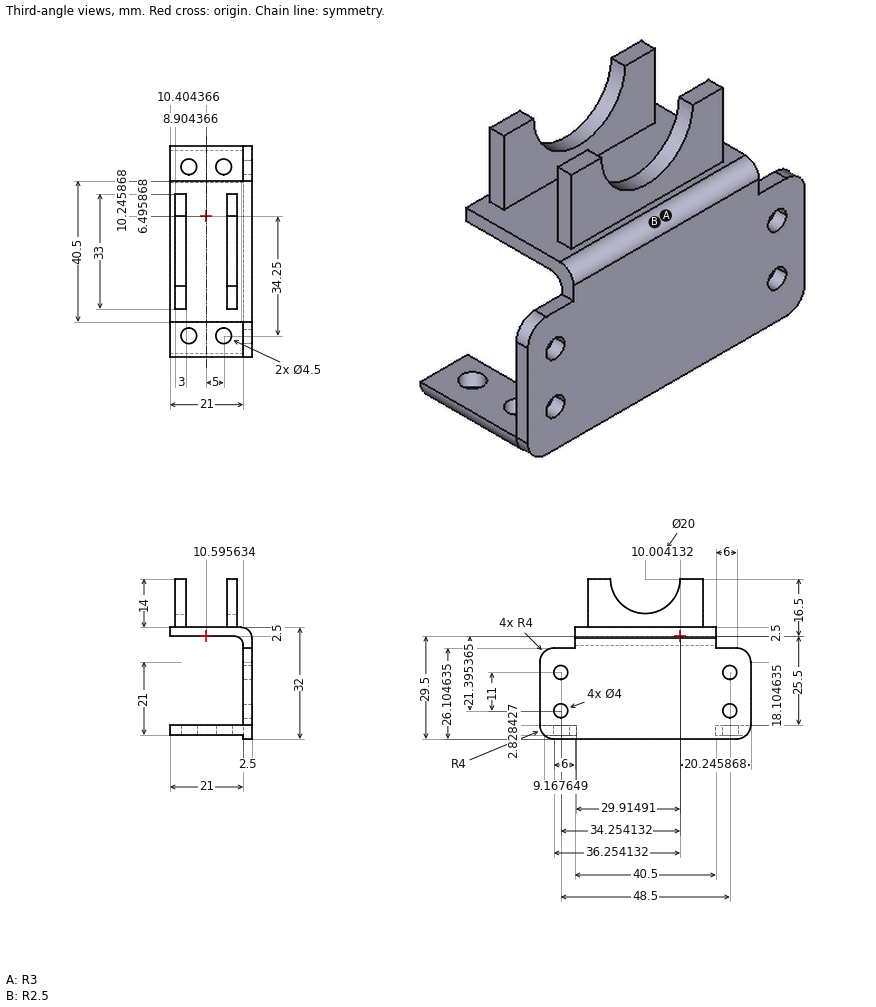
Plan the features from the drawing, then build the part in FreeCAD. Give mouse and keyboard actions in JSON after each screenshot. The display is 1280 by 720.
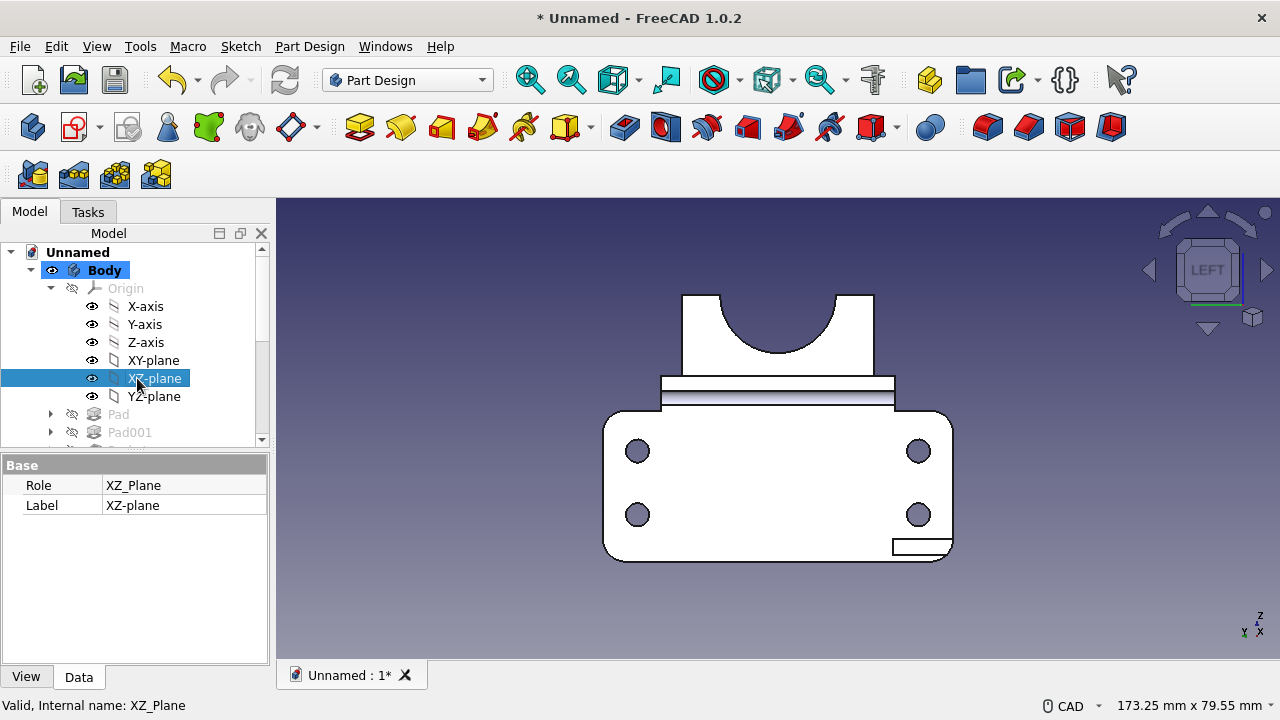
{"action": "left_click", "coordinate": [290, 128]}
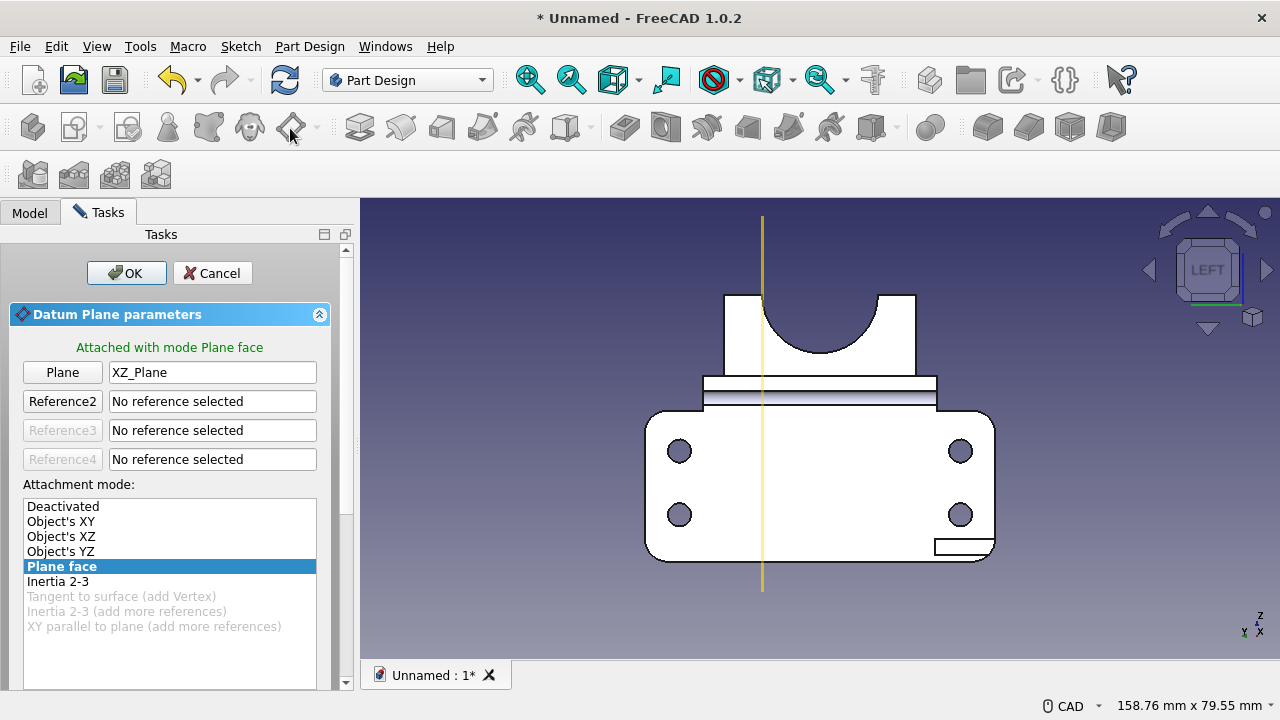
{"action": "scroll", "coordinate": [346, 467], "scroll_direction": "down", "scroll_amount": 4}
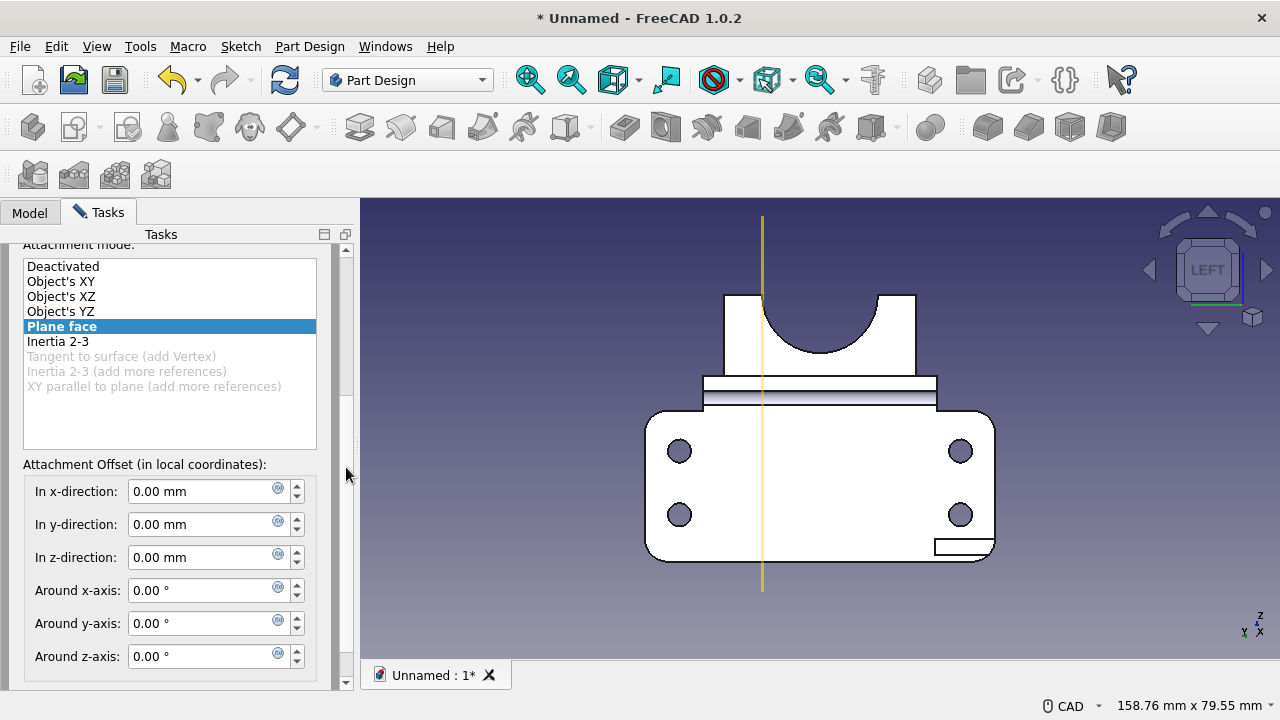
{"action": "triple_click", "coordinate": [210, 558]}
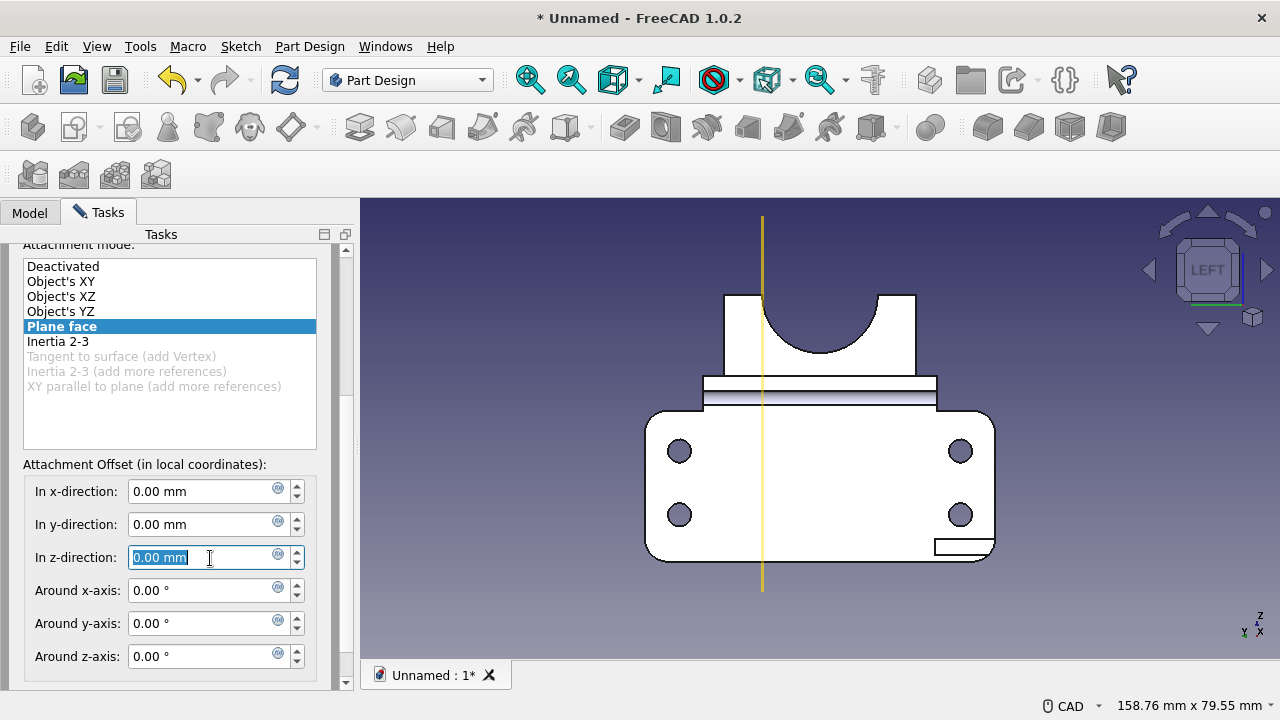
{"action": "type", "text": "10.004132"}
{"action": "key", "text": "Tab"}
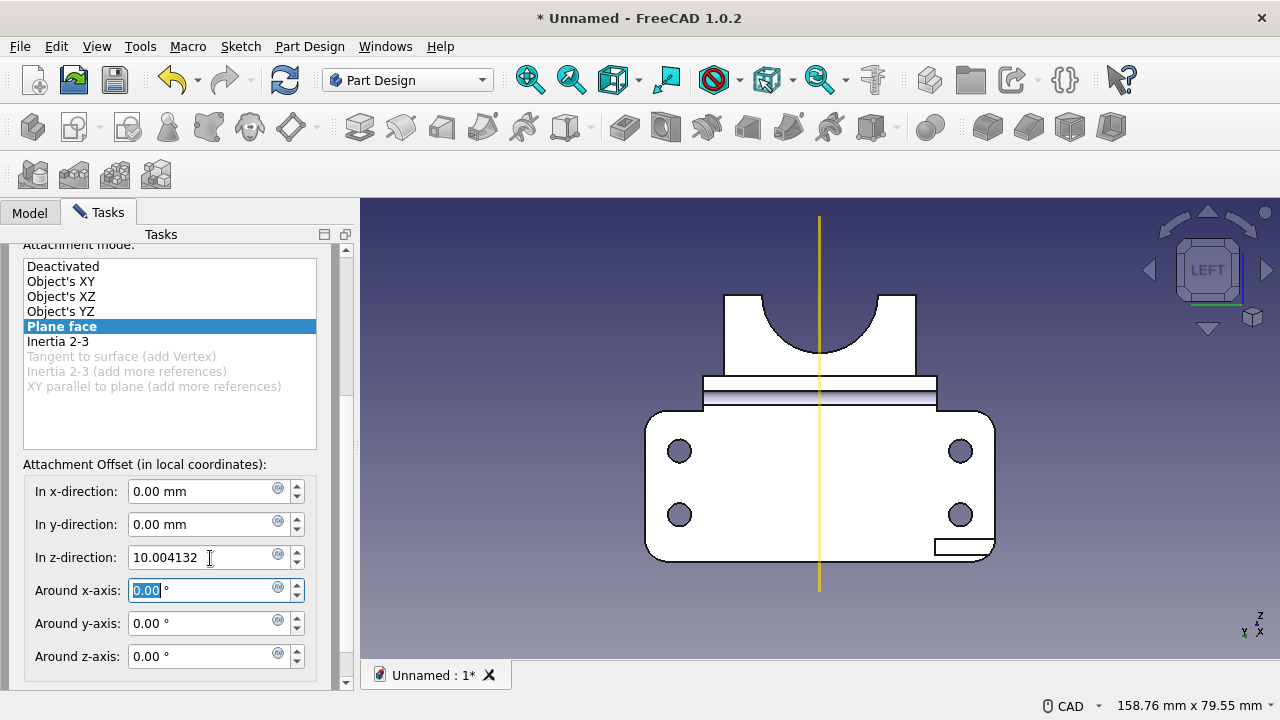
{"action": "scroll", "coordinate": [346, 467], "scroll_direction": "up", "scroll_amount": 5}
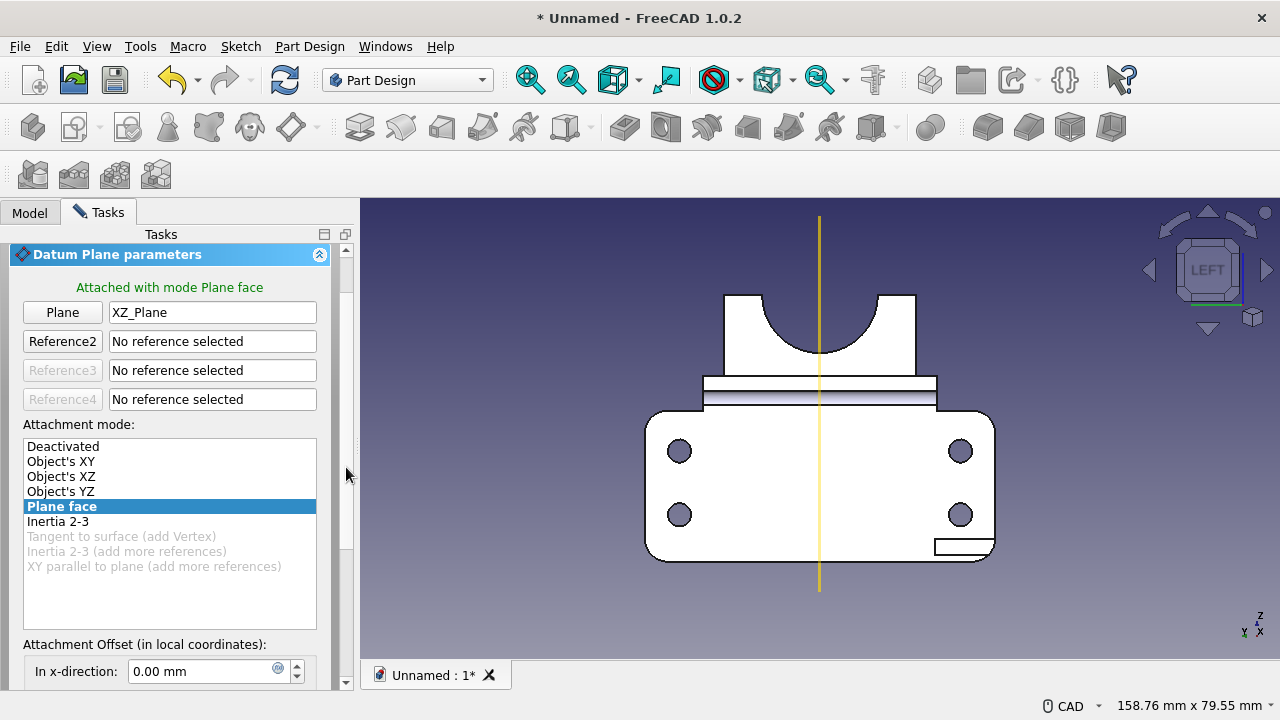
{"action": "left_click", "coordinate": [127, 273]}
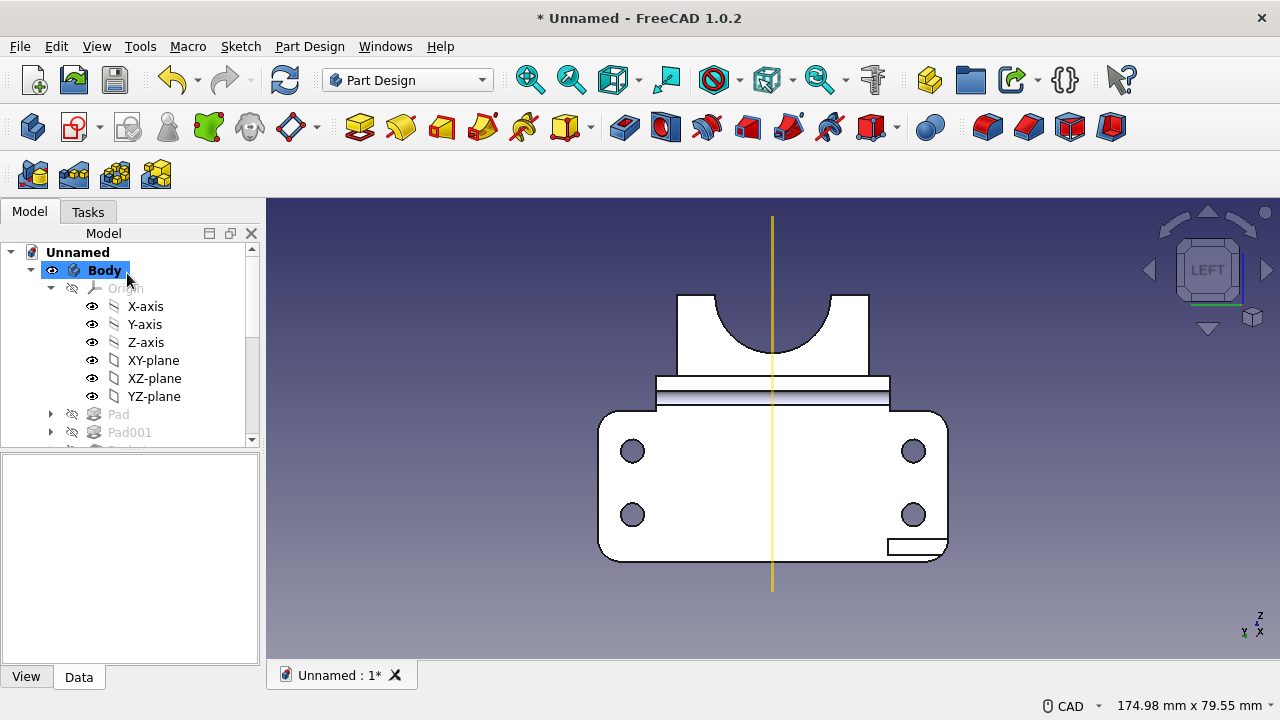
{"action": "scroll", "coordinate": [101, 338], "scroll_direction": "down", "scroll_amount": 3}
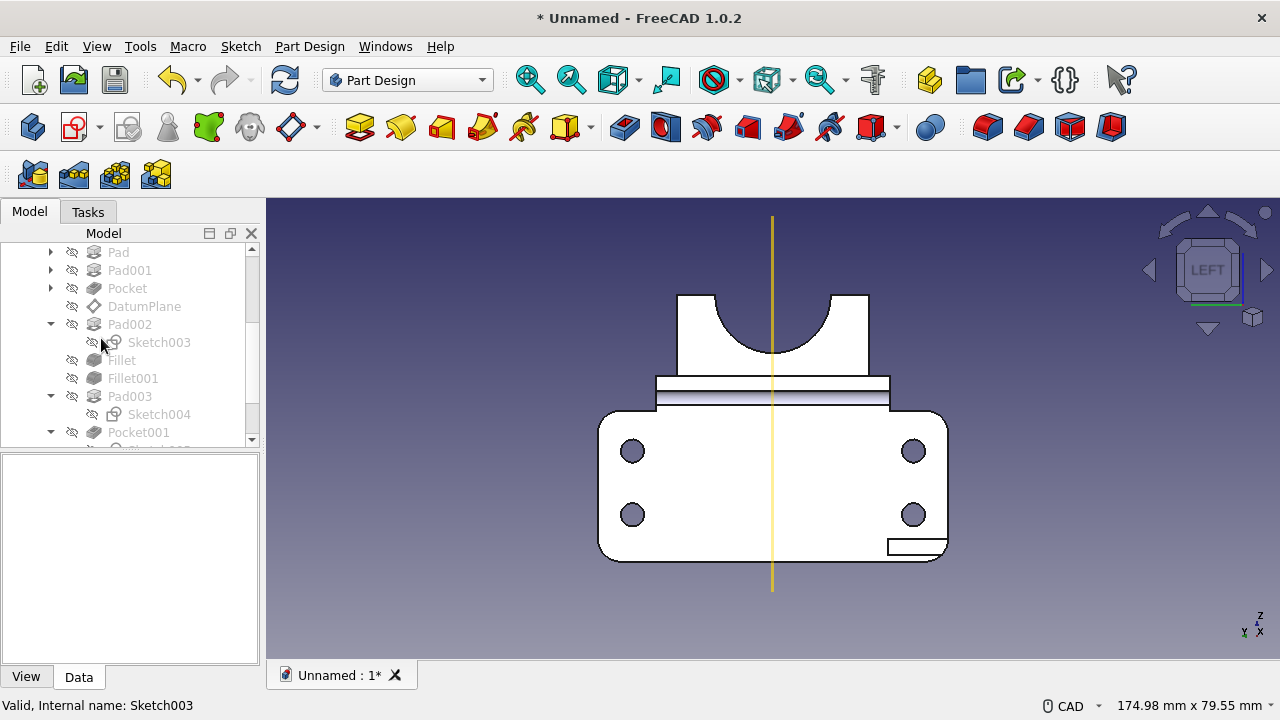
{"action": "scroll", "coordinate": [141, 338], "scroll_direction": "up", "scroll_amount": 15}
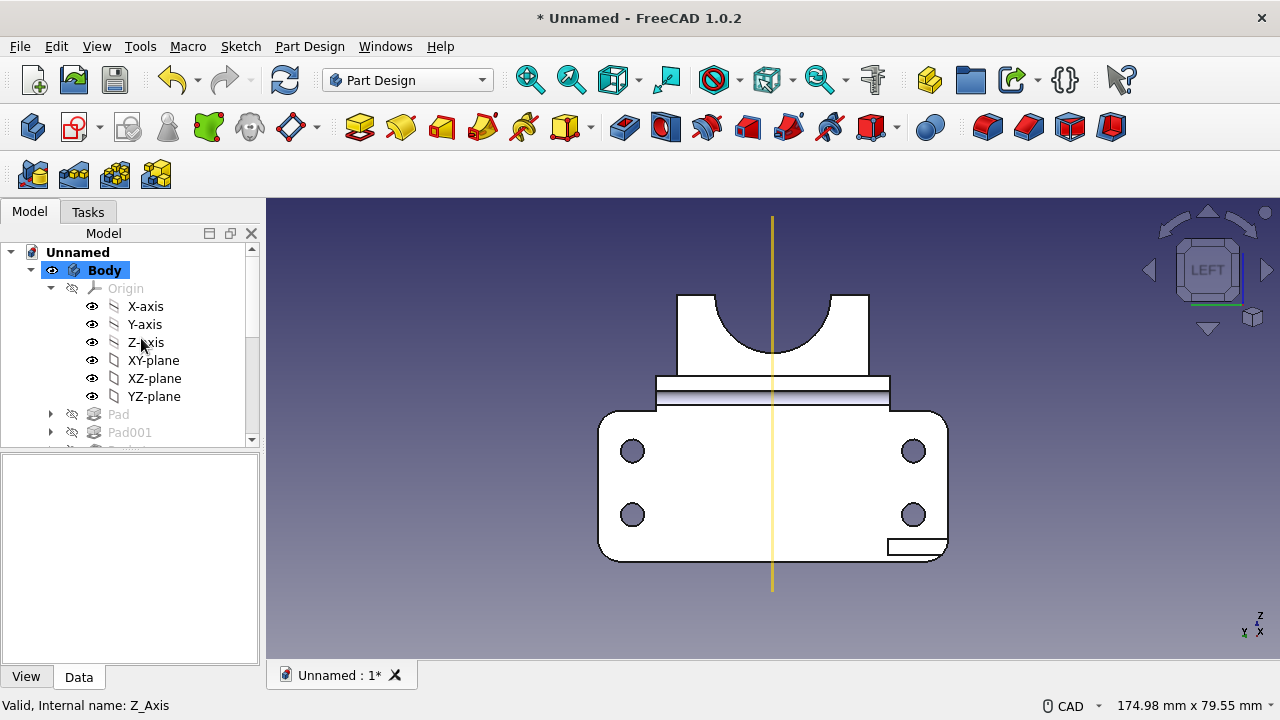
{"action": "scroll", "coordinate": [101, 338], "scroll_direction": "down", "scroll_amount": 6}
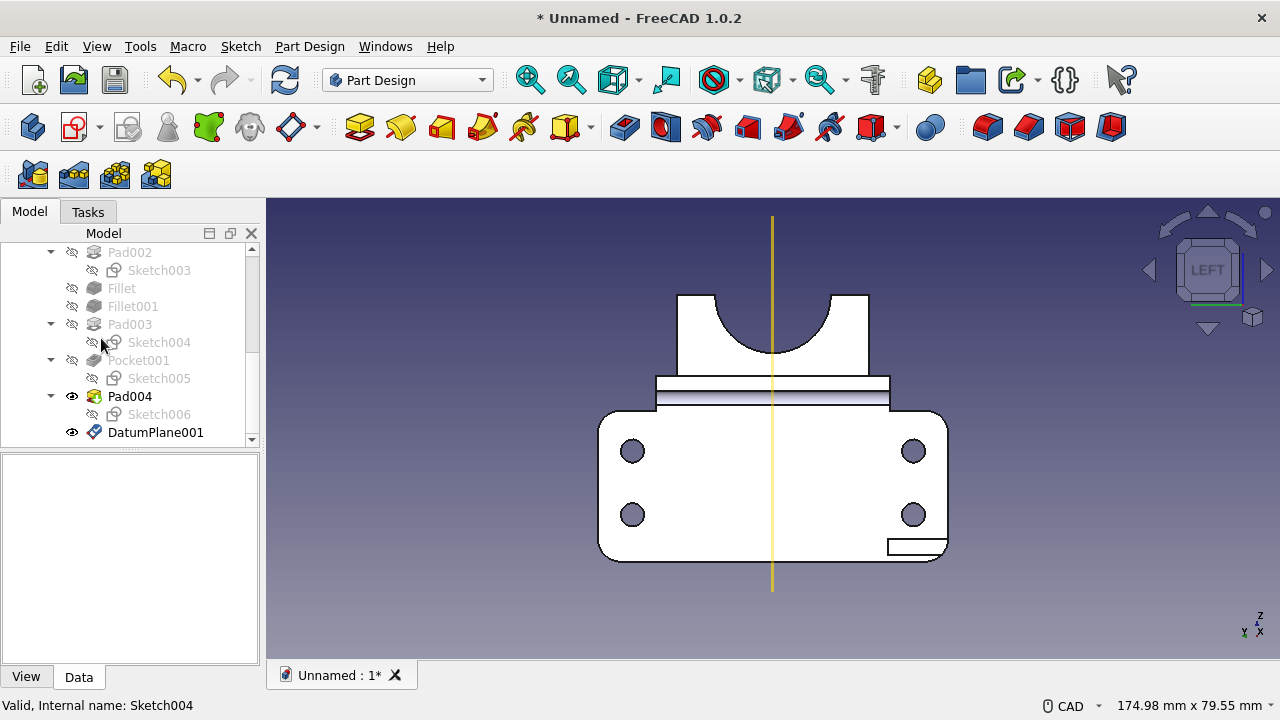
{"action": "left_click", "coordinate": [117, 396]}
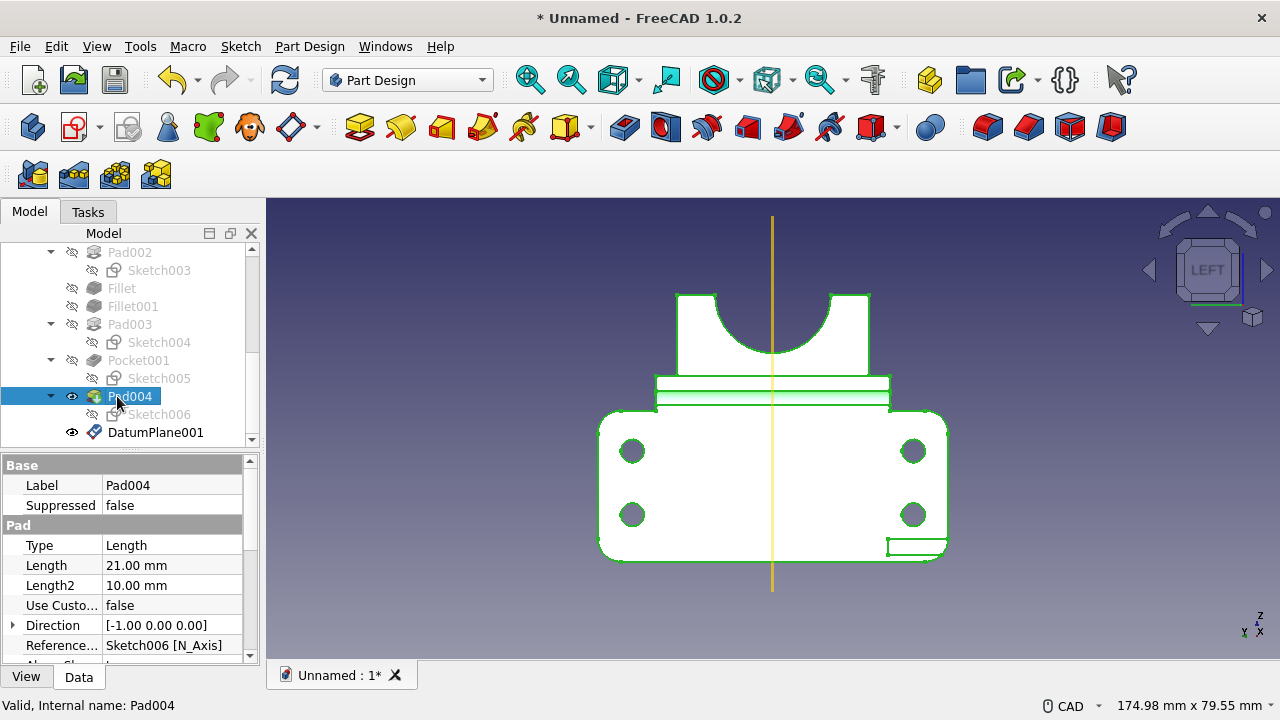
{"action": "left_click", "coordinate": [33, 174]}